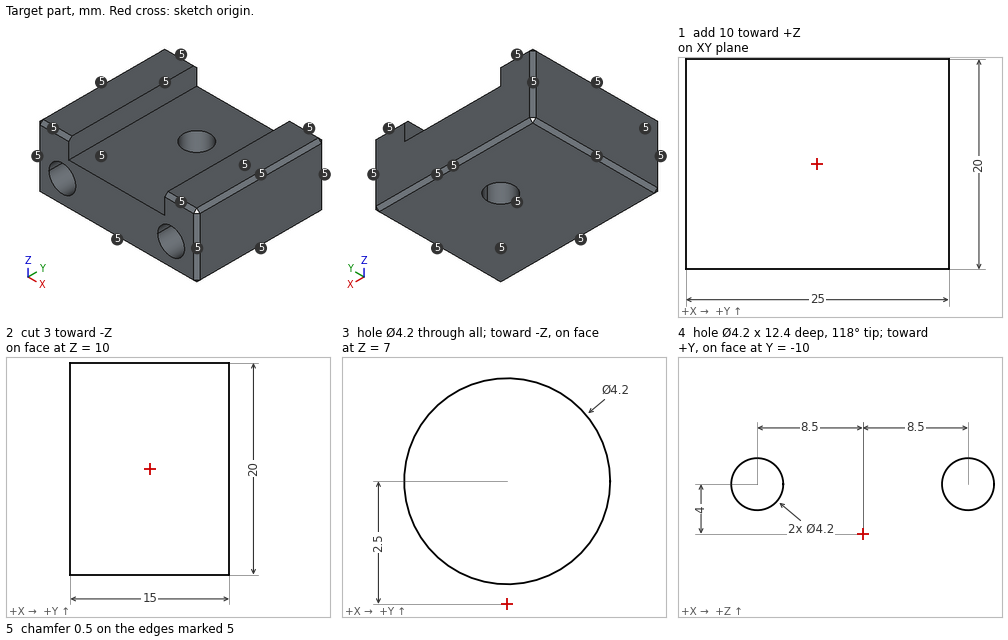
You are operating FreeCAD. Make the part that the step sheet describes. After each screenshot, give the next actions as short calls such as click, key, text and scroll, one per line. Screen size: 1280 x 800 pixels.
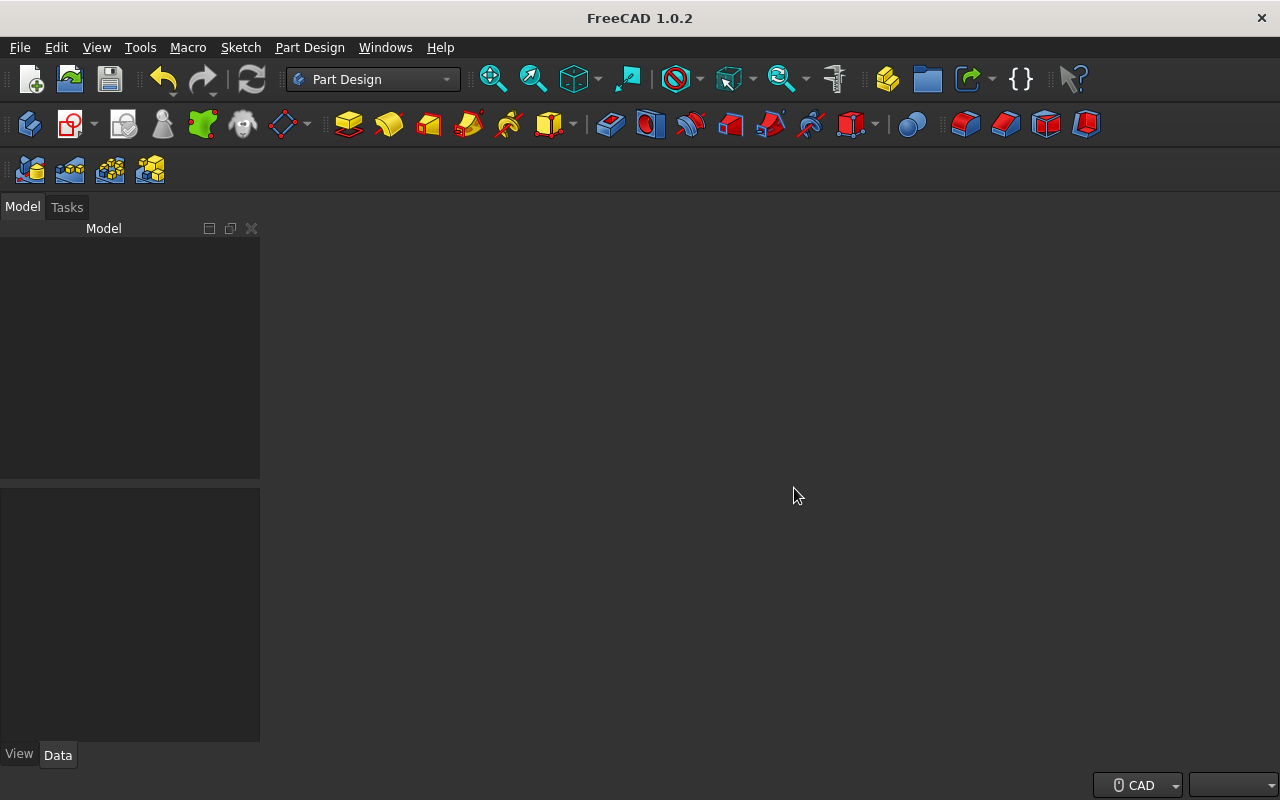
key(ctrl+n)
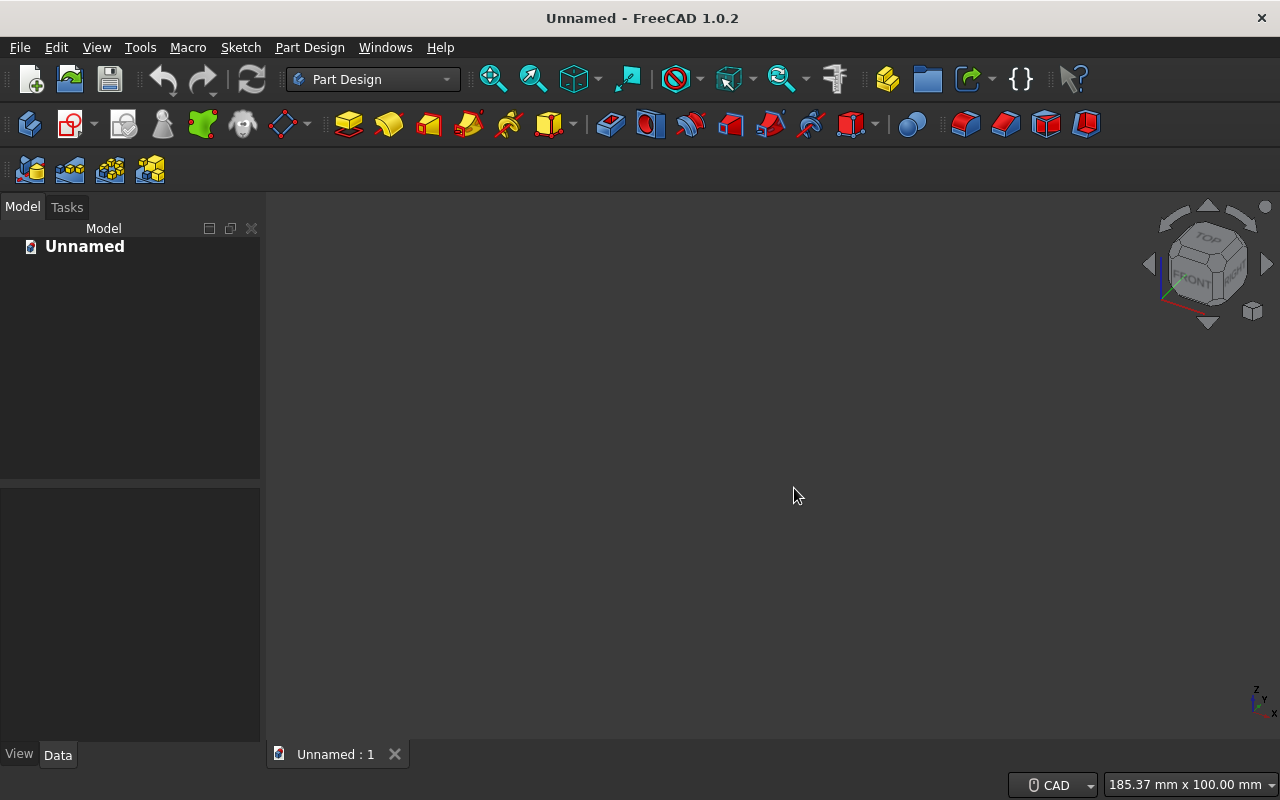
click(70, 124)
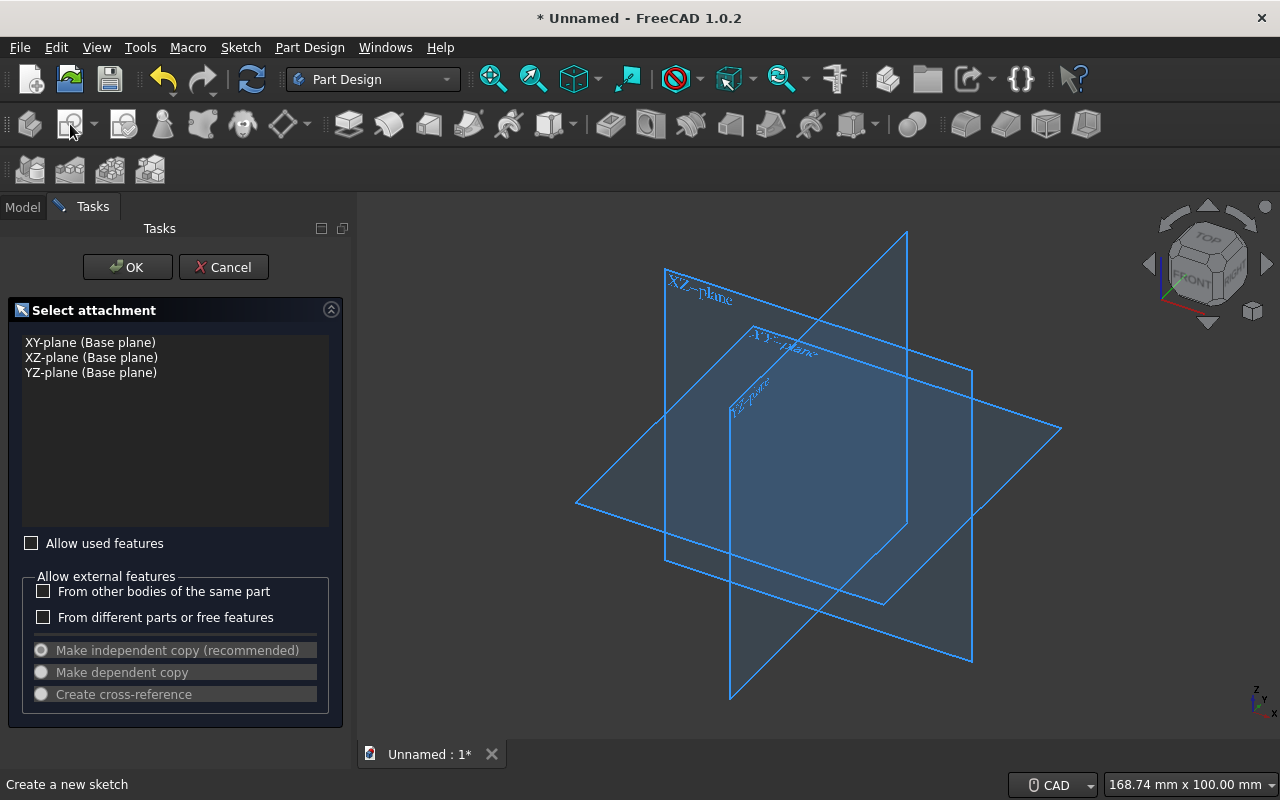
click(82, 342)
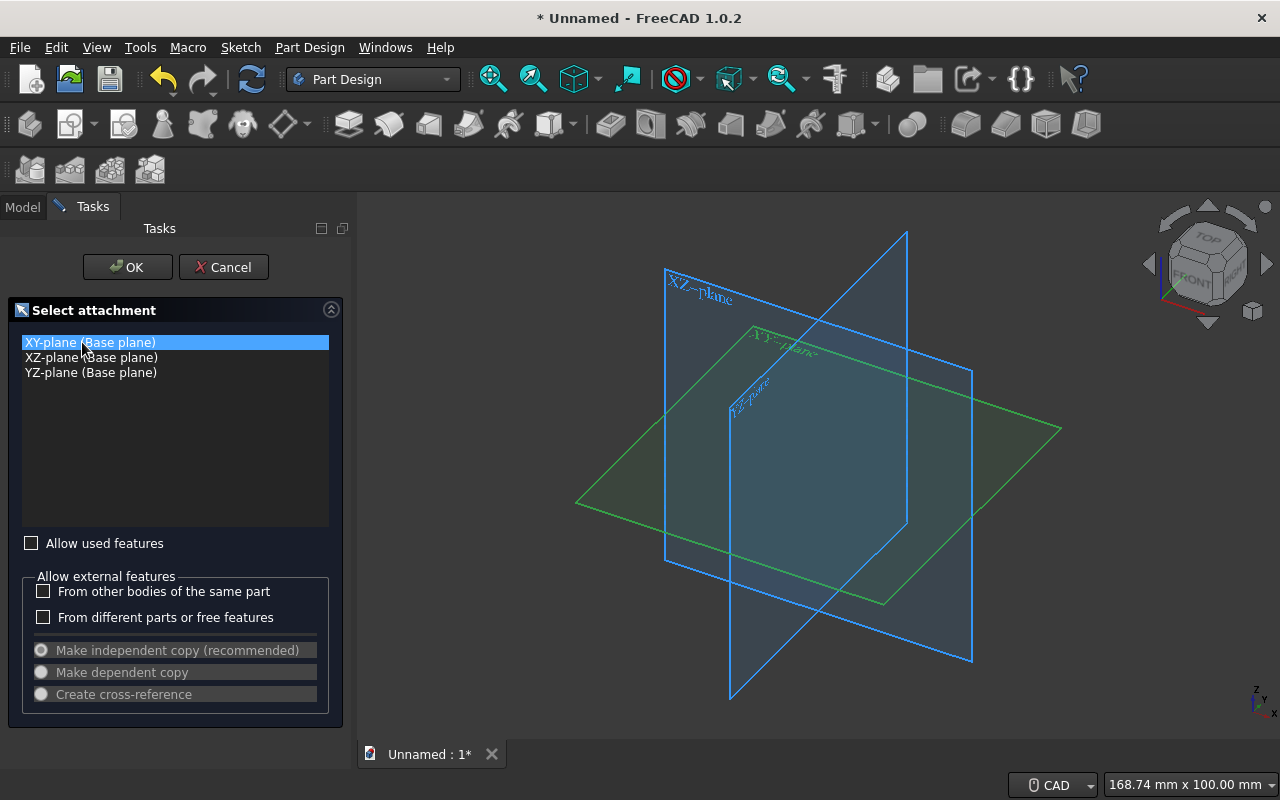
click(128, 267)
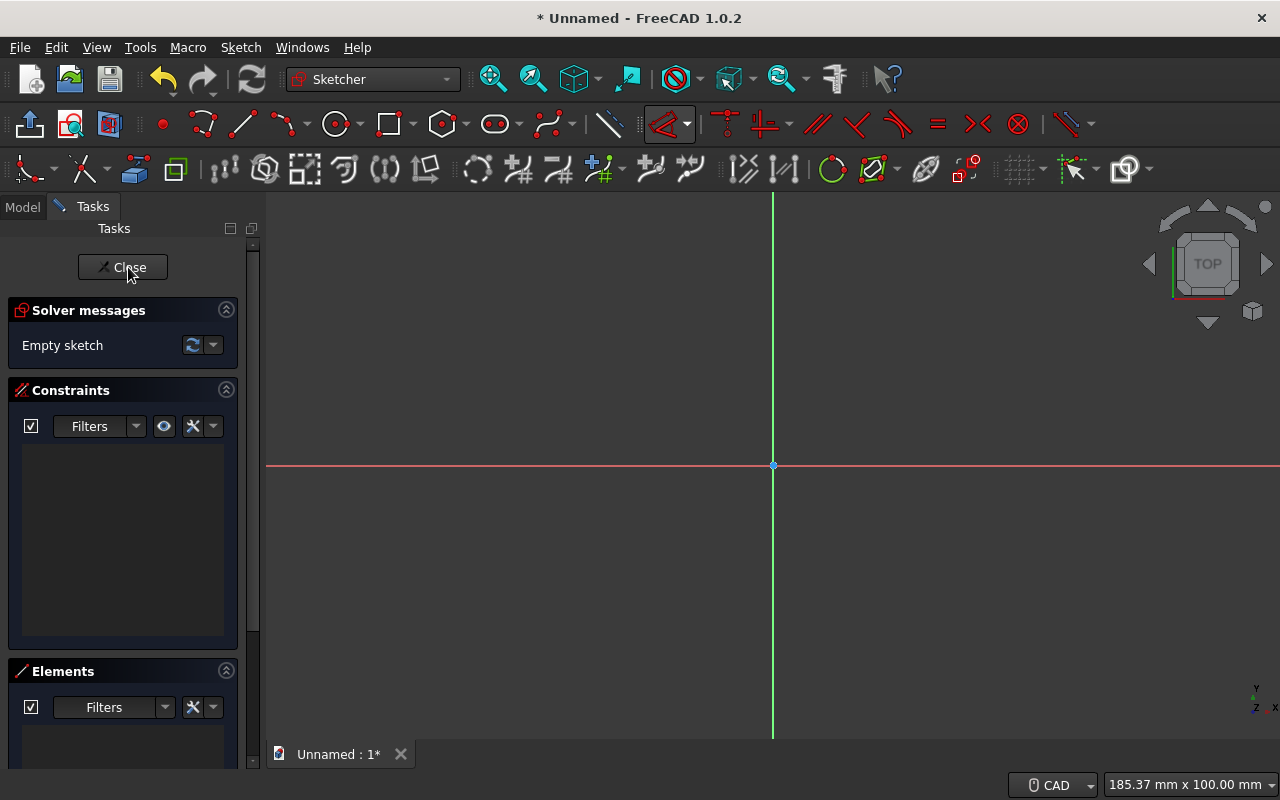
scroll(803, 466, up, 6)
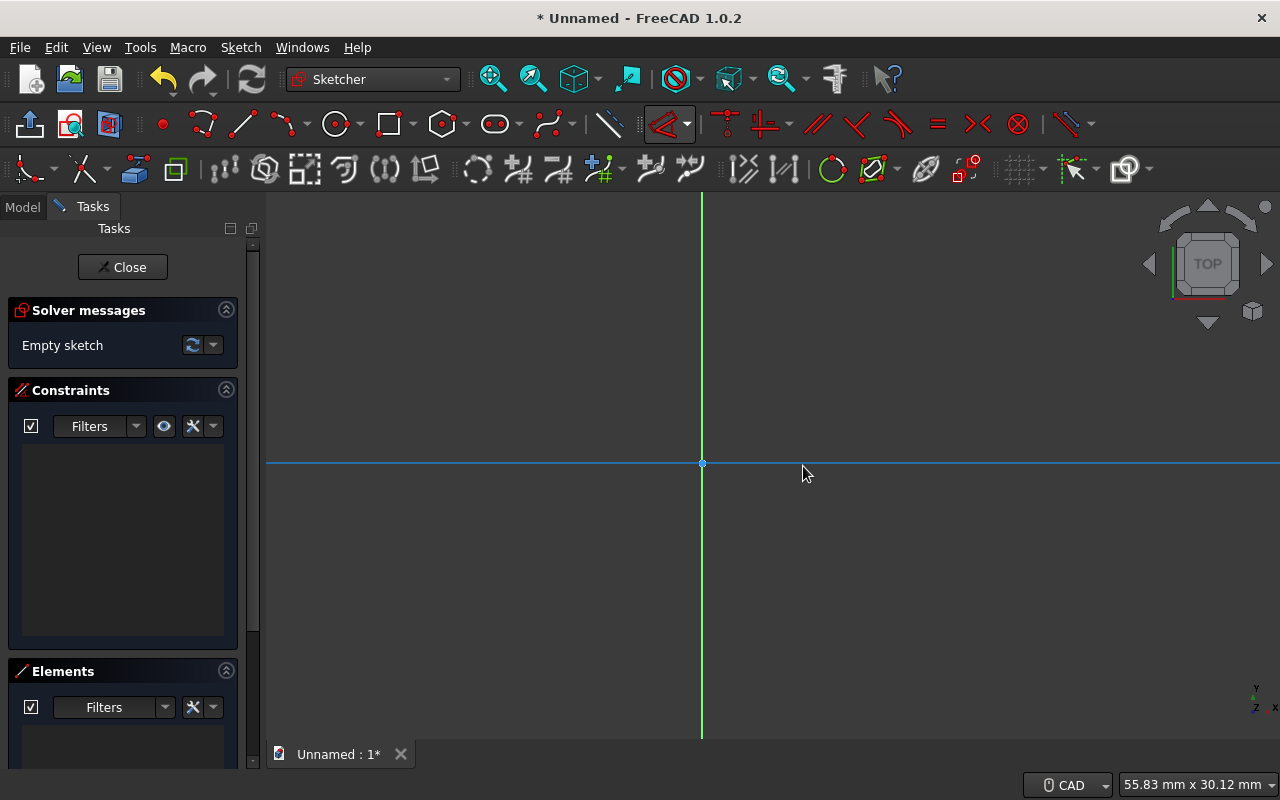
key(g)
key(v)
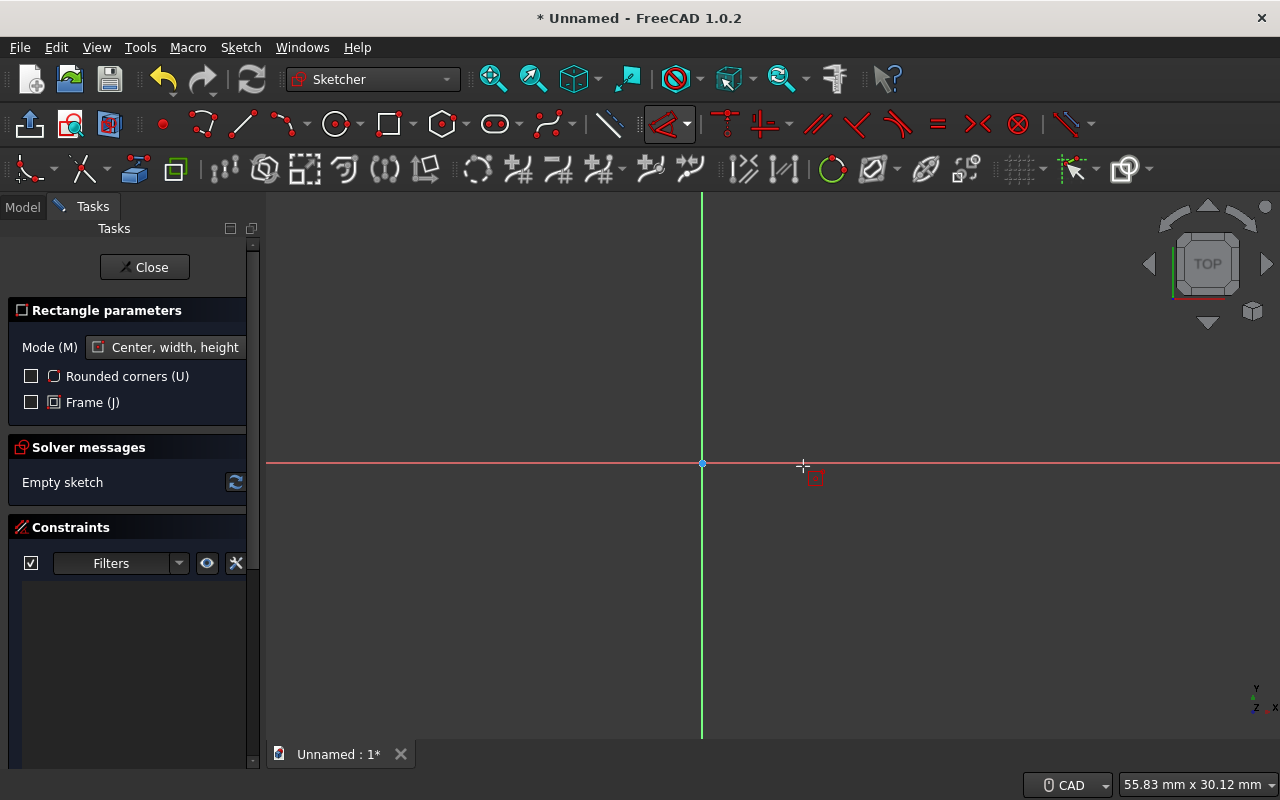
click(702, 463)
move(929, 282)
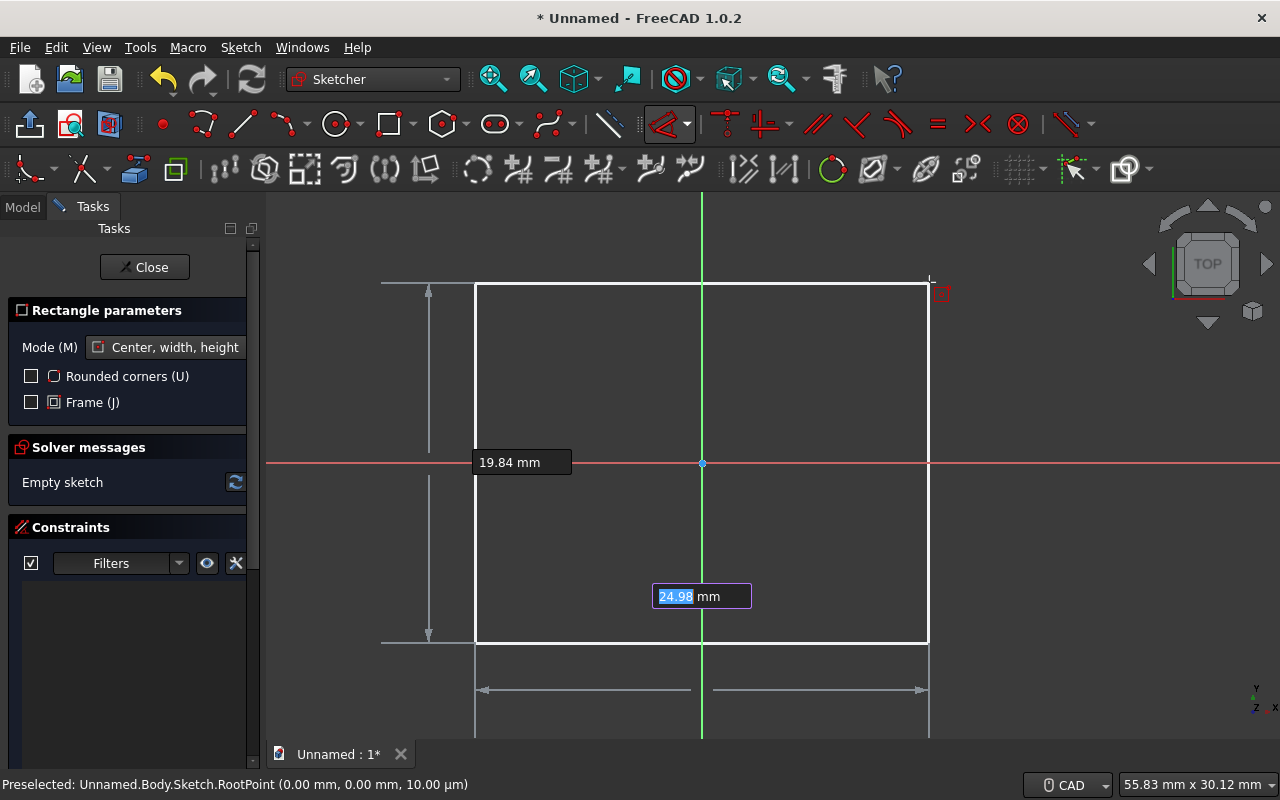
text(25)
key(Tab)
text(20)
key(Return)
key(Escape)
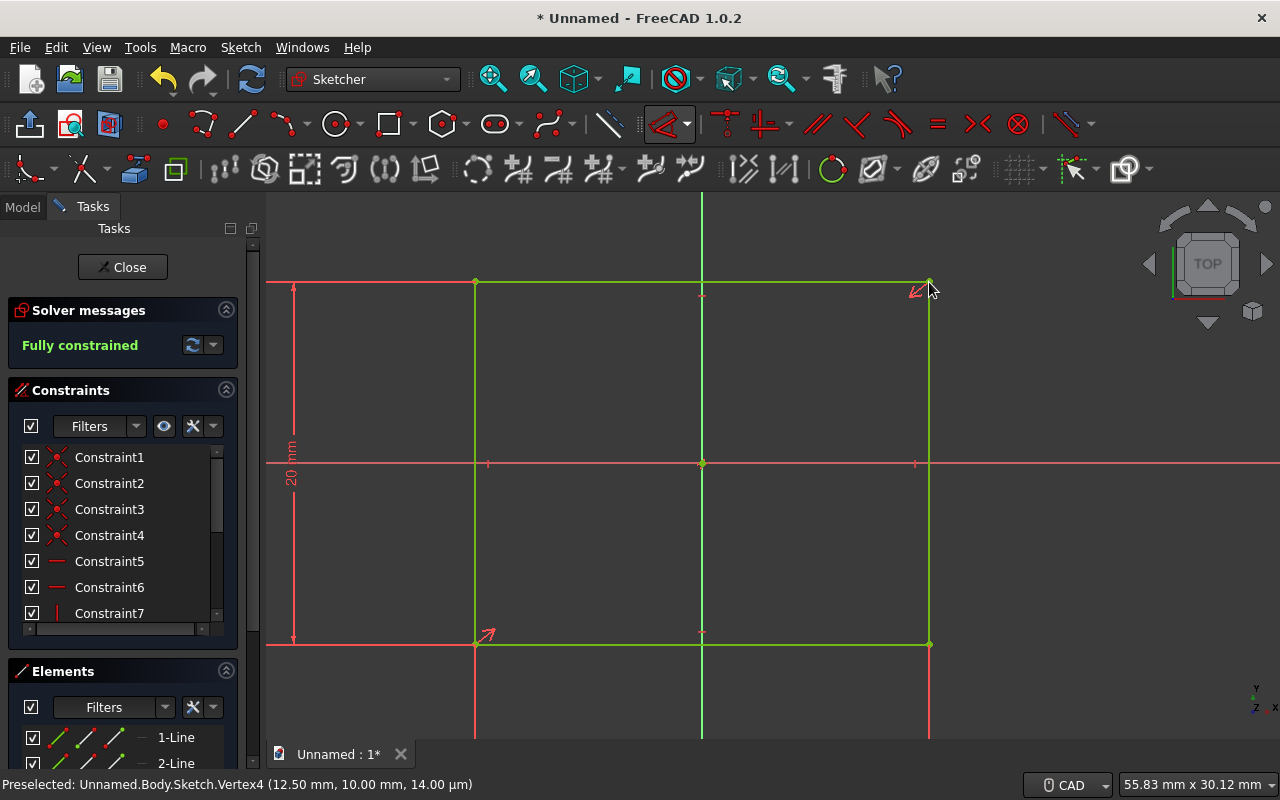
click(123, 267)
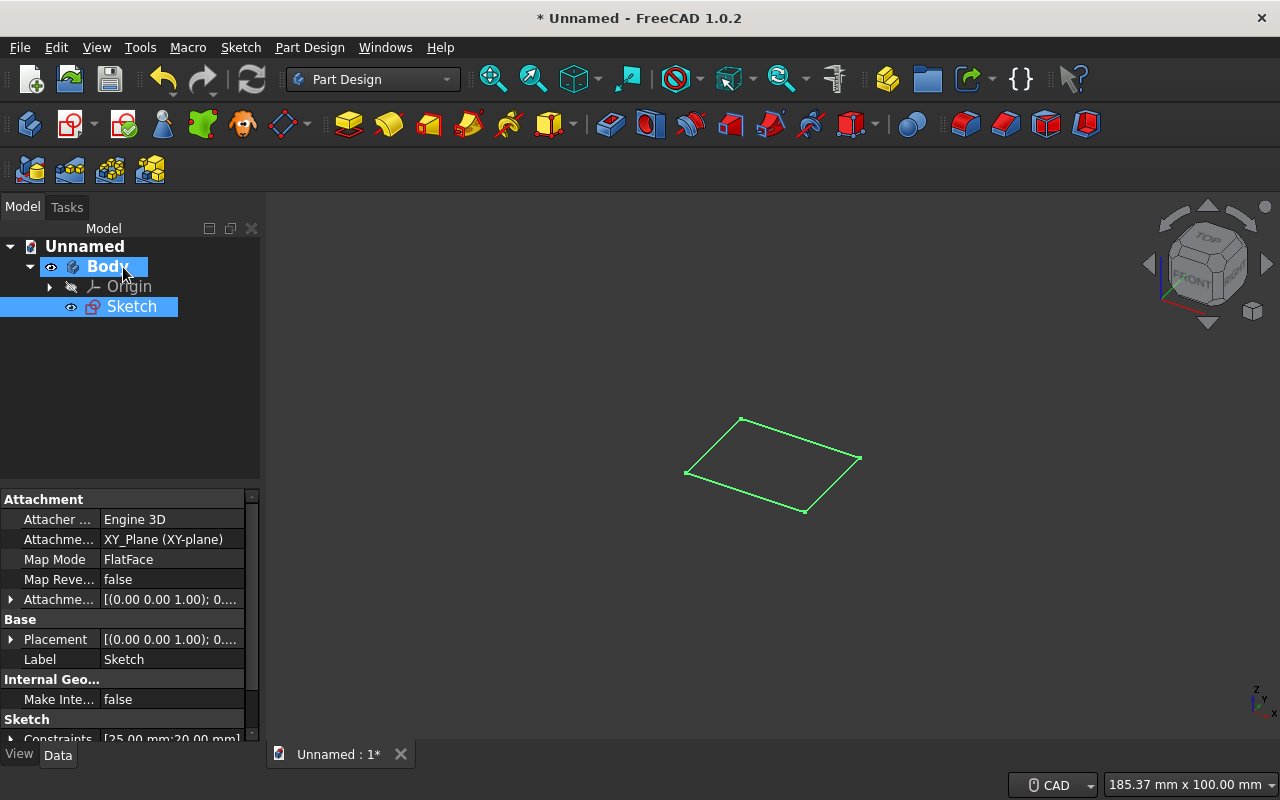
click(350, 124)